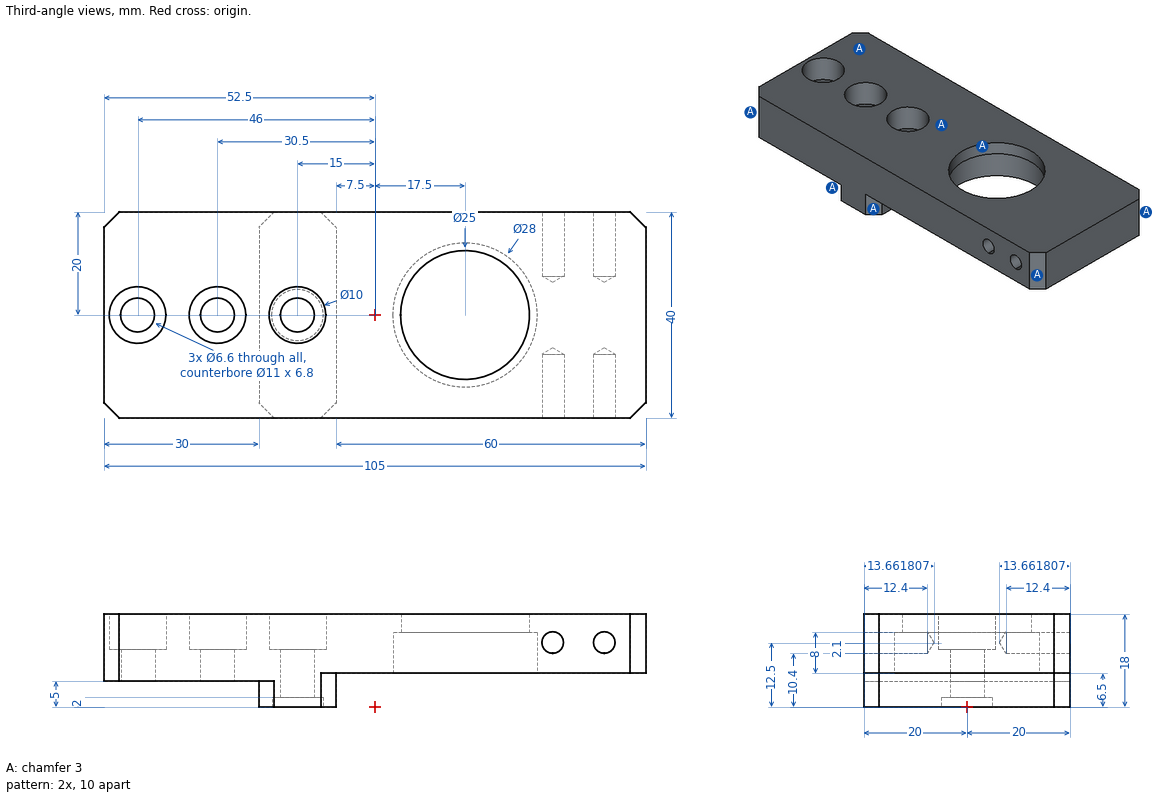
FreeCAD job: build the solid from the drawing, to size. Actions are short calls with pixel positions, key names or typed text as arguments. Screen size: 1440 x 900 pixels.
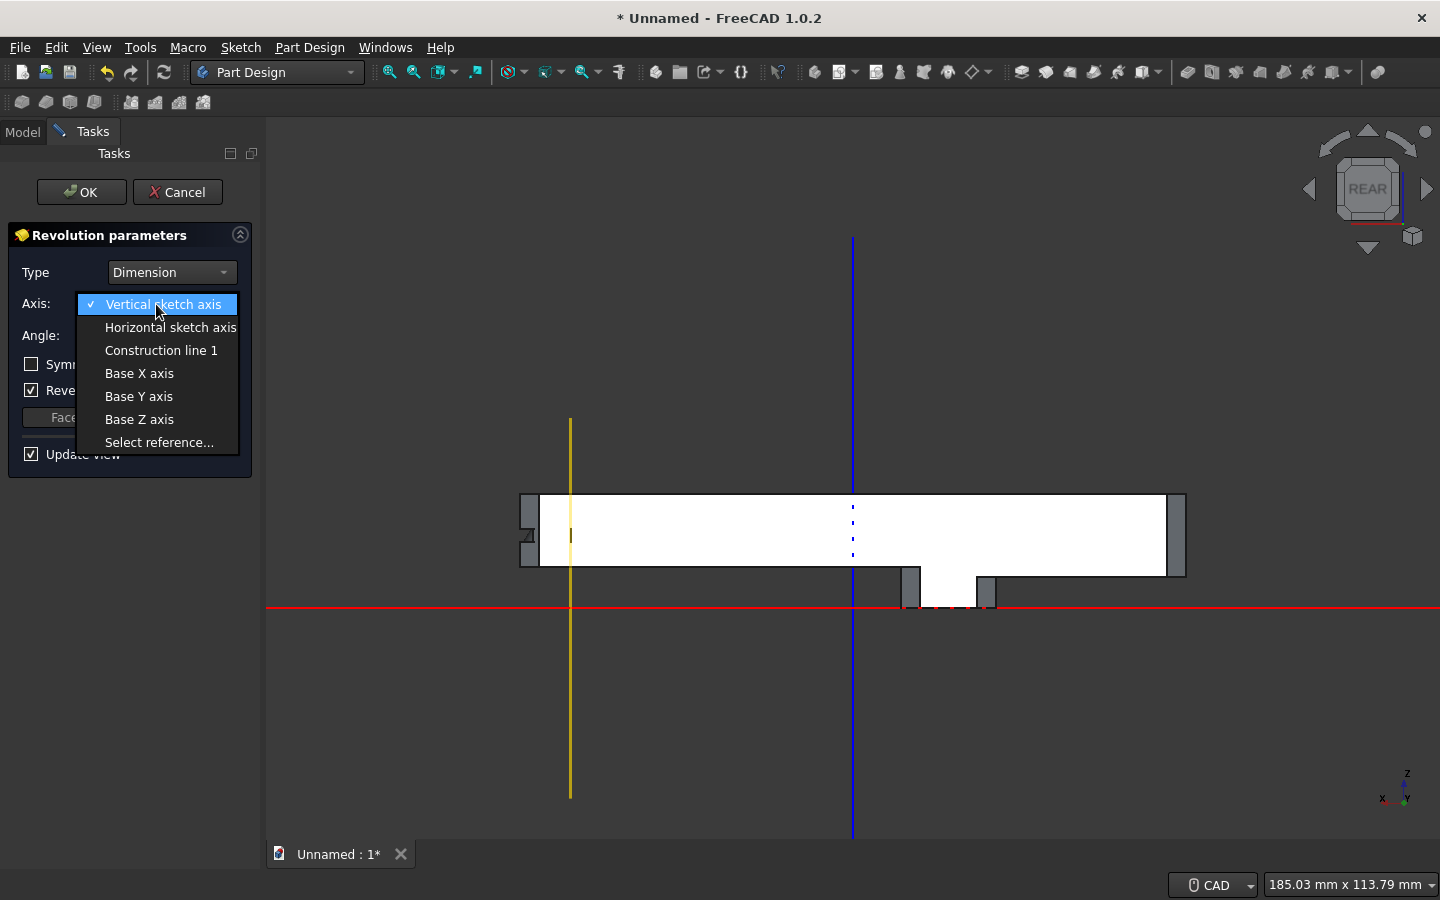
click(156, 350)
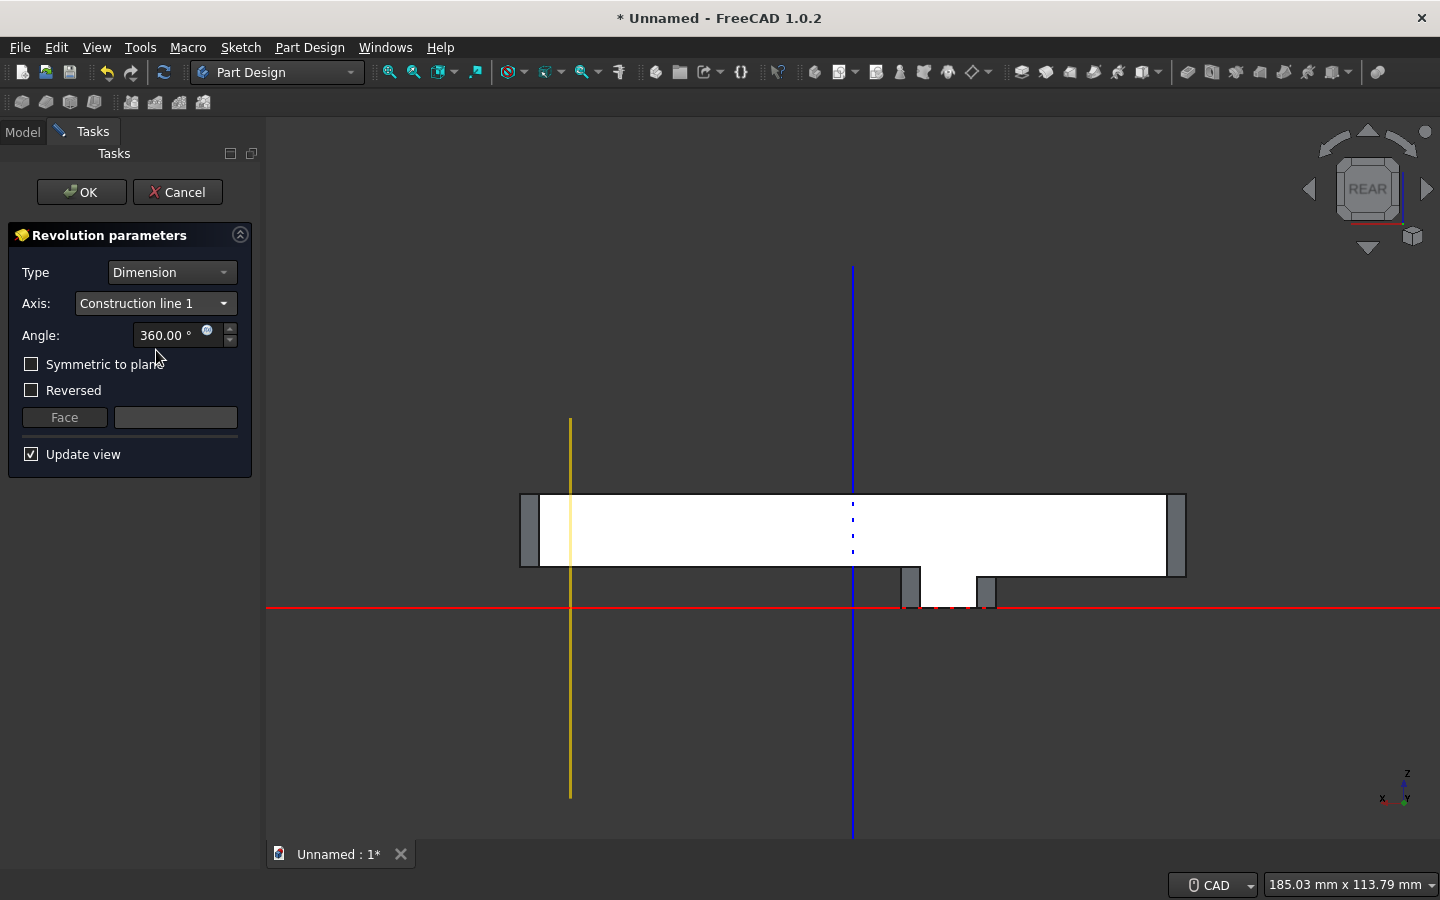
click(82, 192)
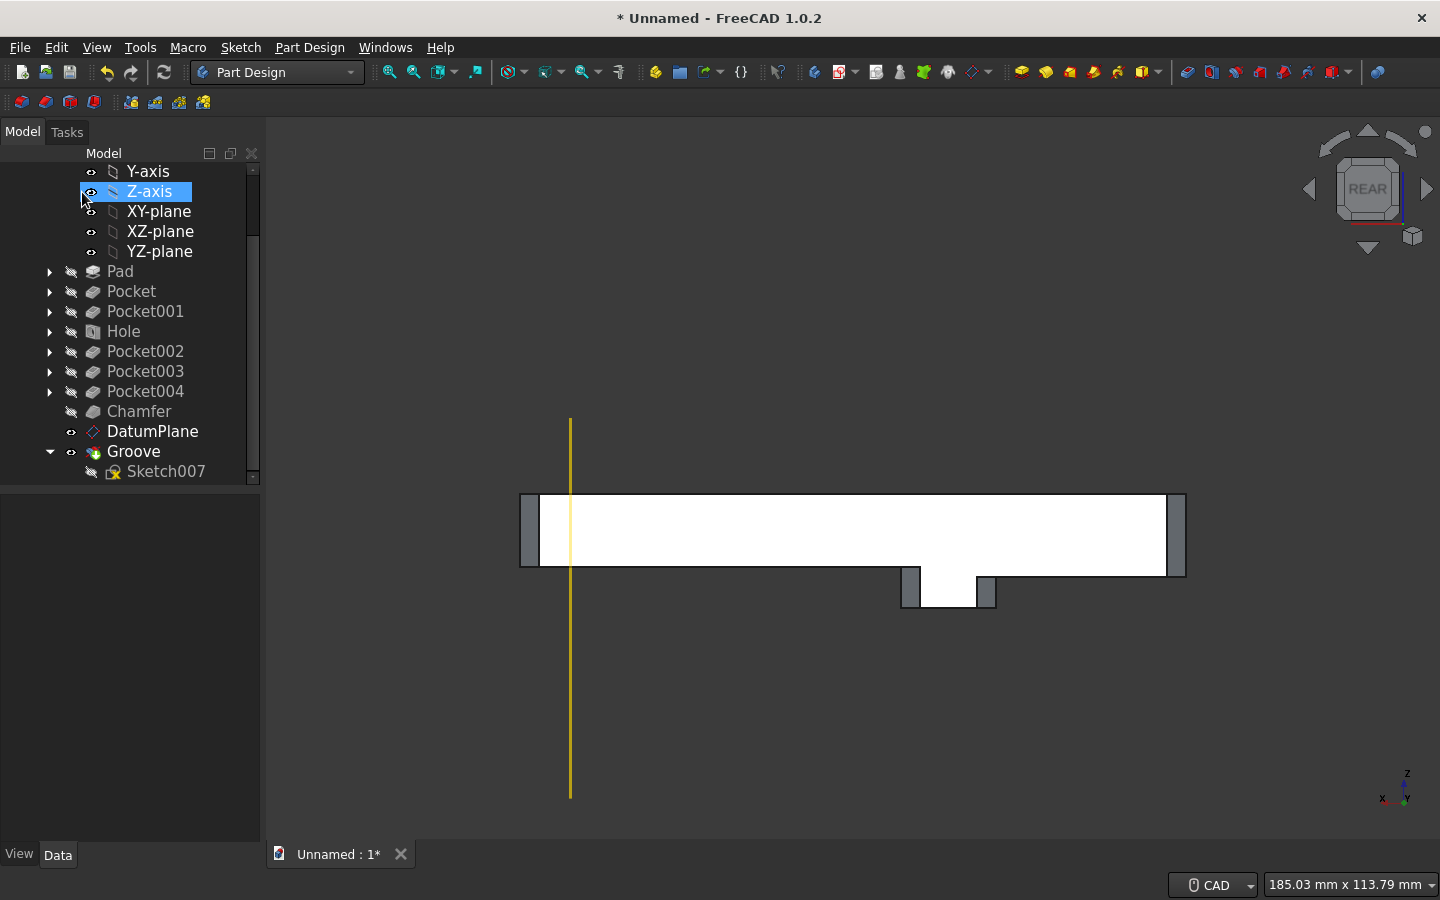
click(116, 432)
key(space)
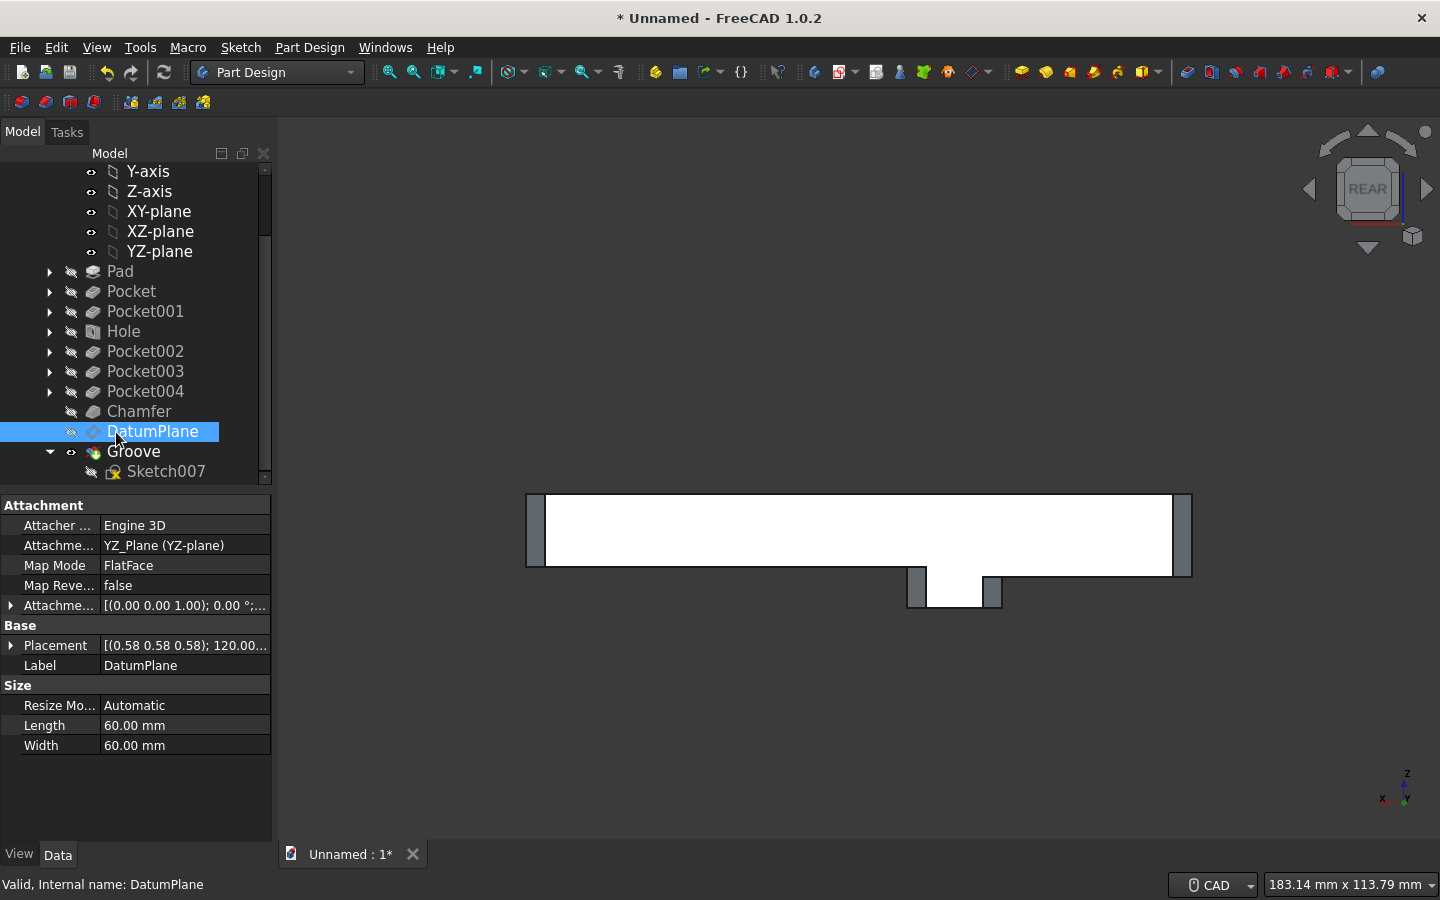
click(116, 452)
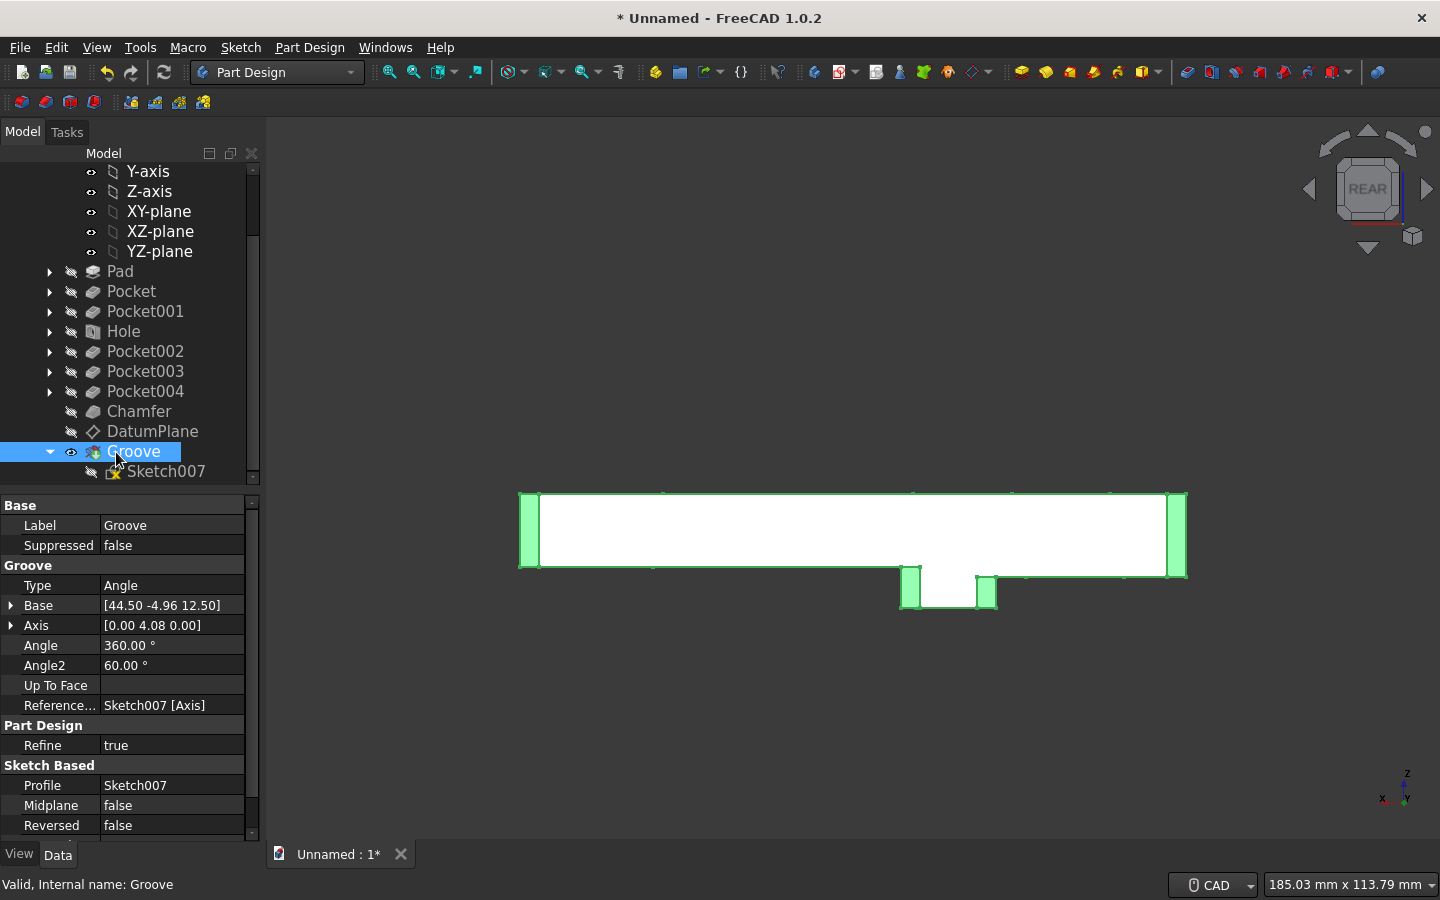
click(156, 102)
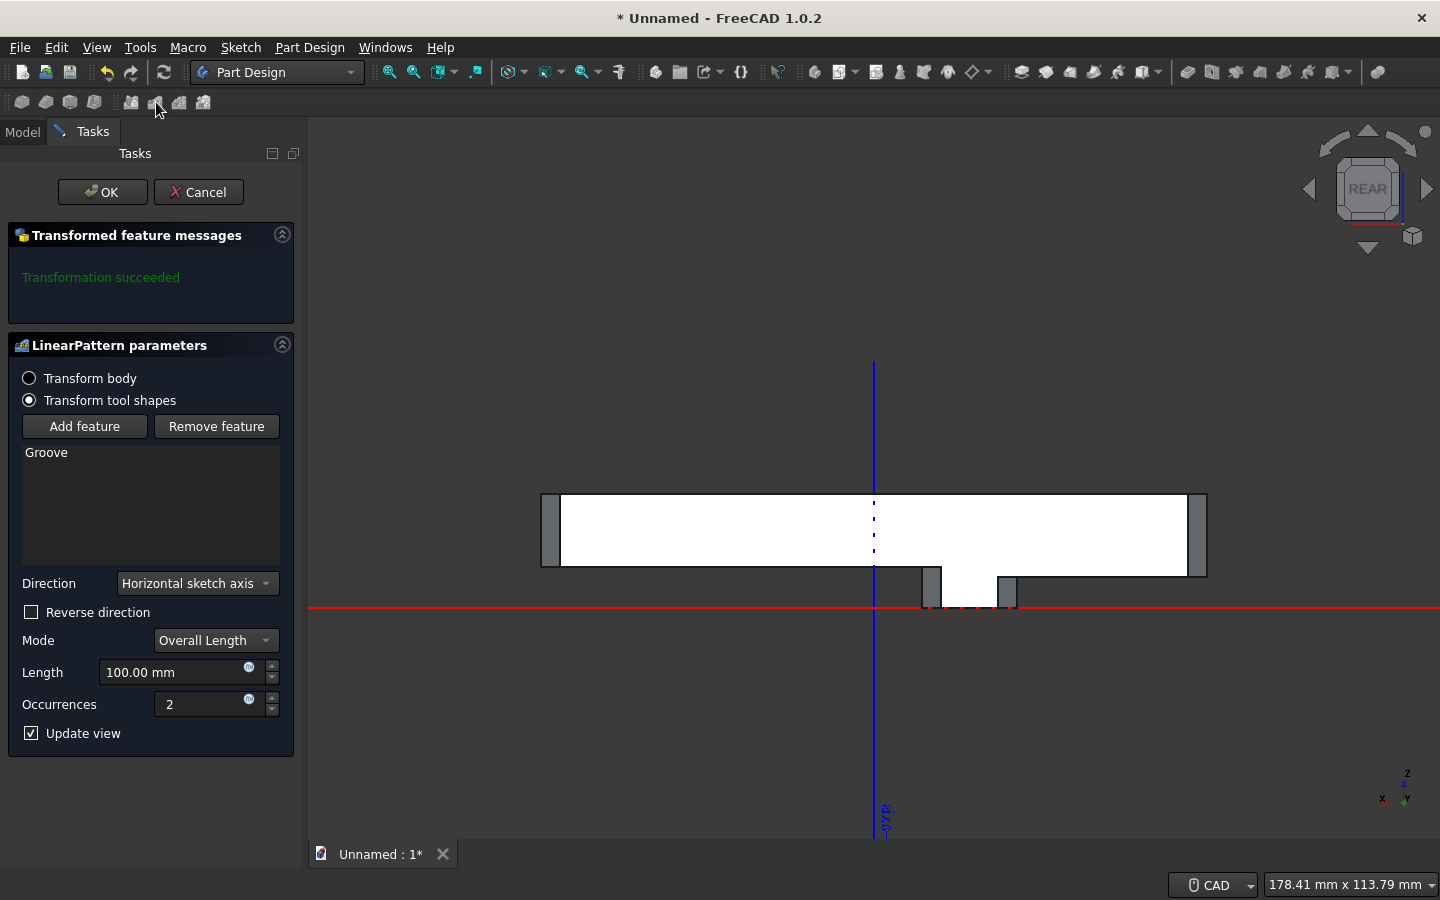
click(198, 584)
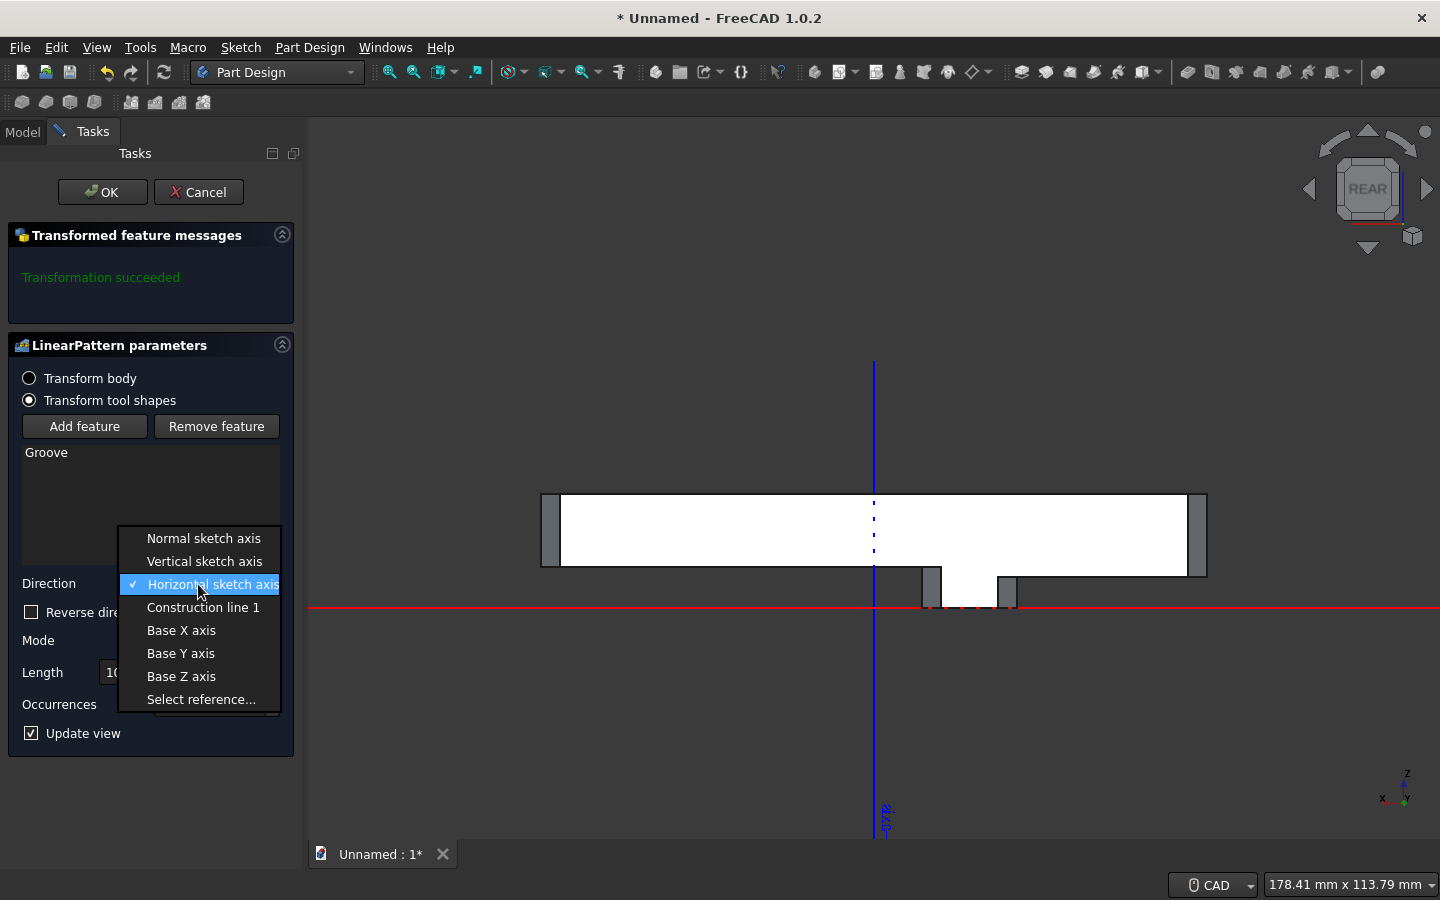
click(198, 630)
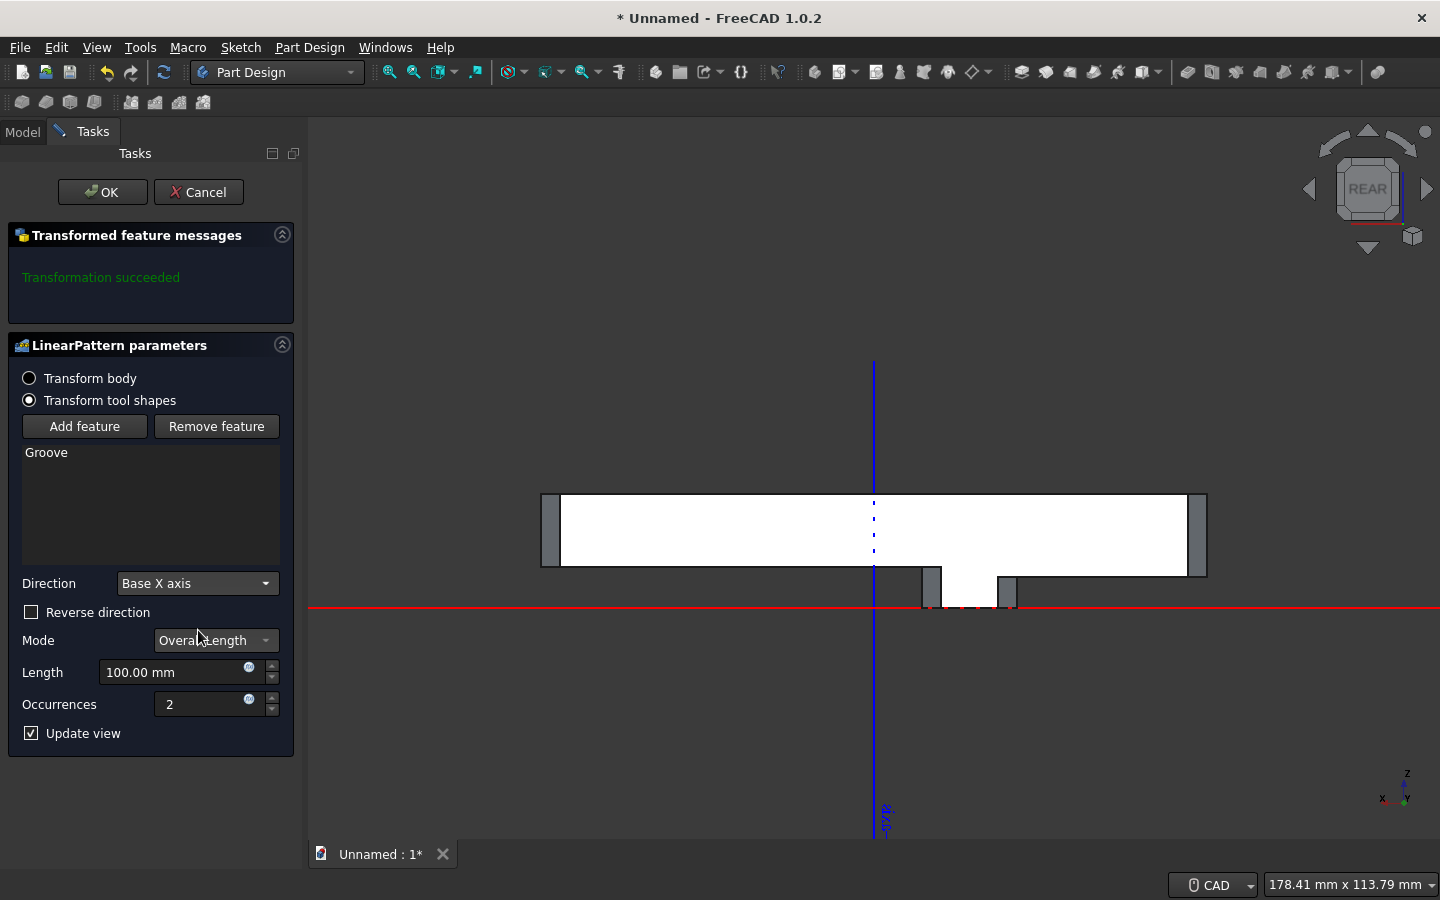
click(217, 640)